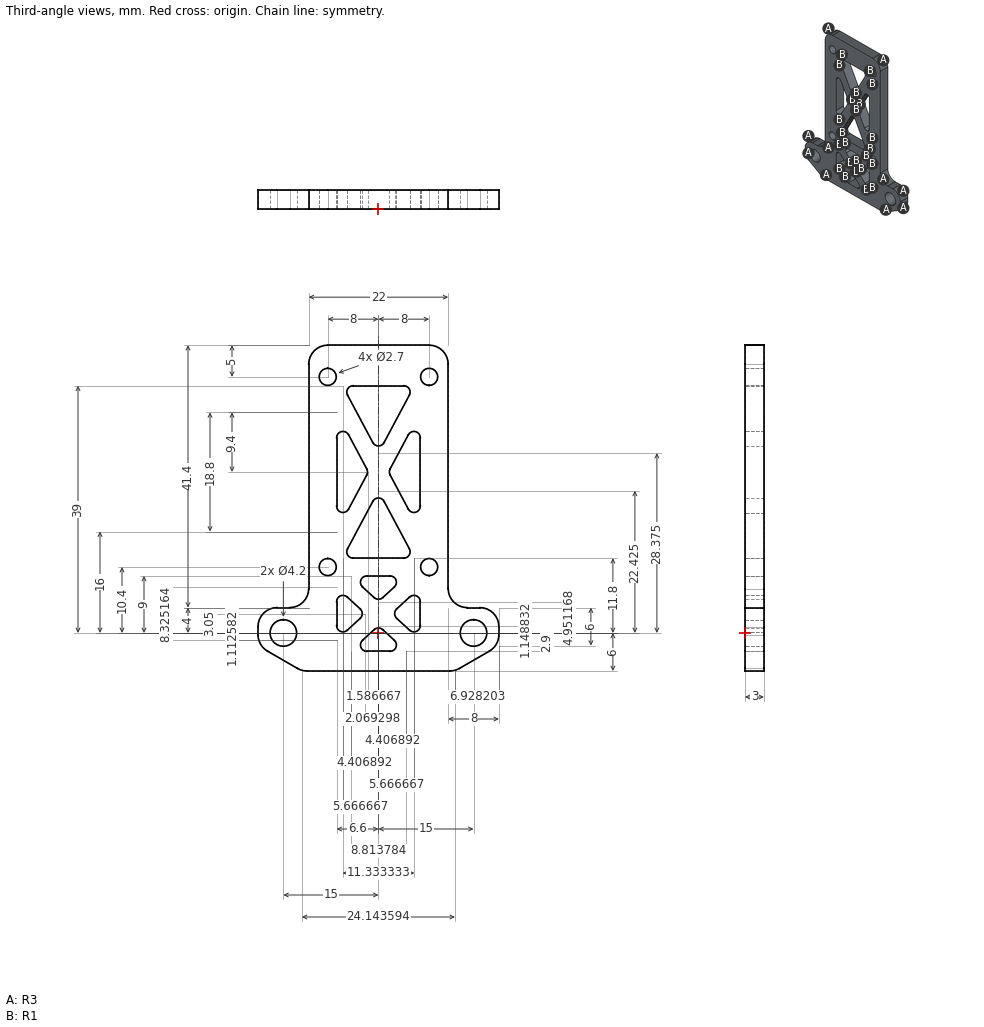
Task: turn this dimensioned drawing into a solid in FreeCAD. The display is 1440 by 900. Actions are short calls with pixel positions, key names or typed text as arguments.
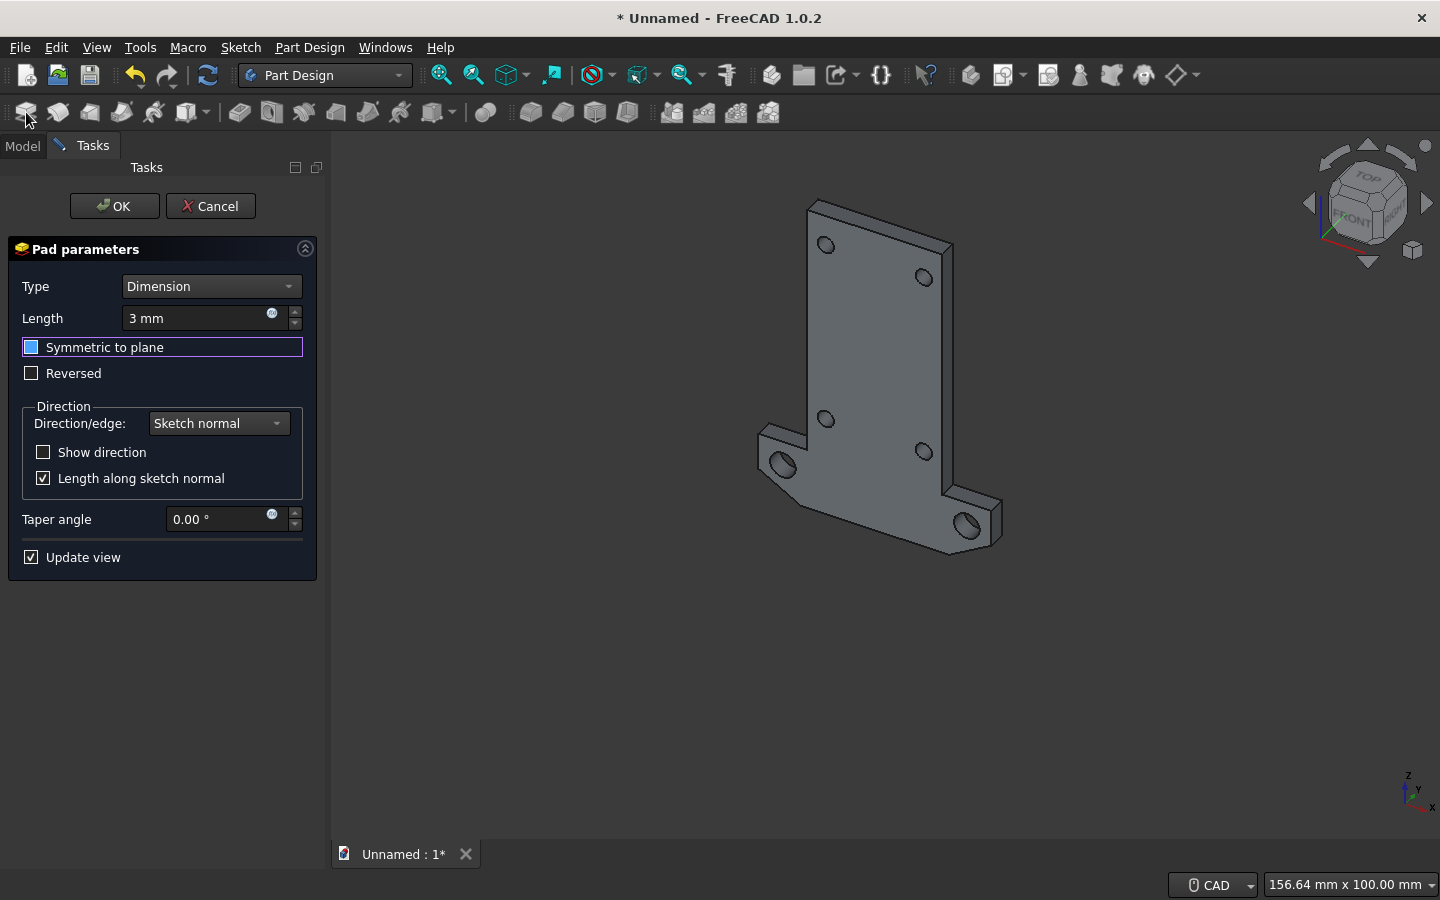
click(30, 373)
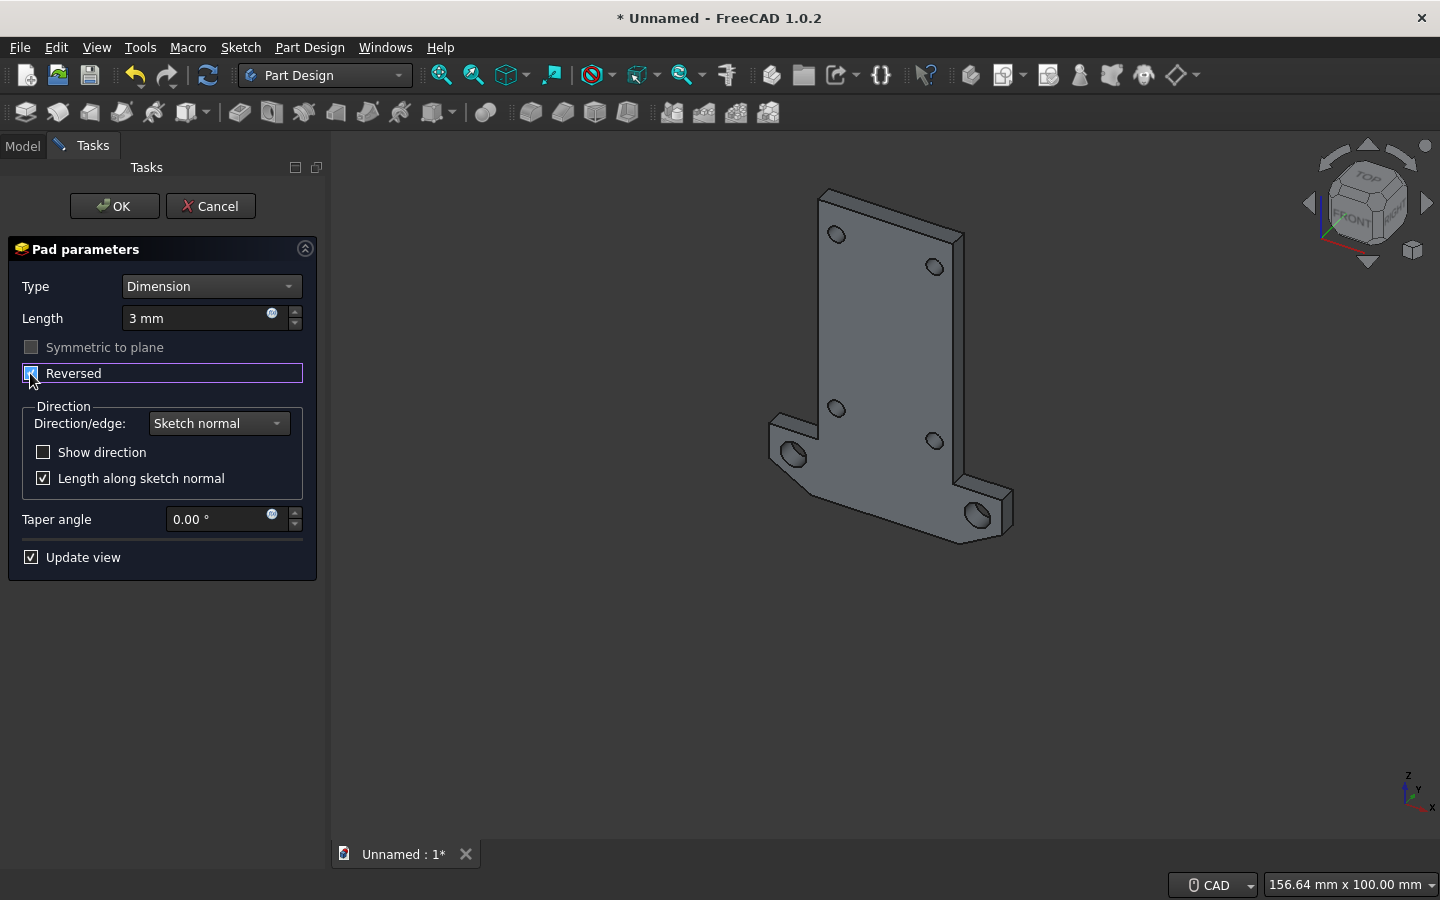
click(115, 206)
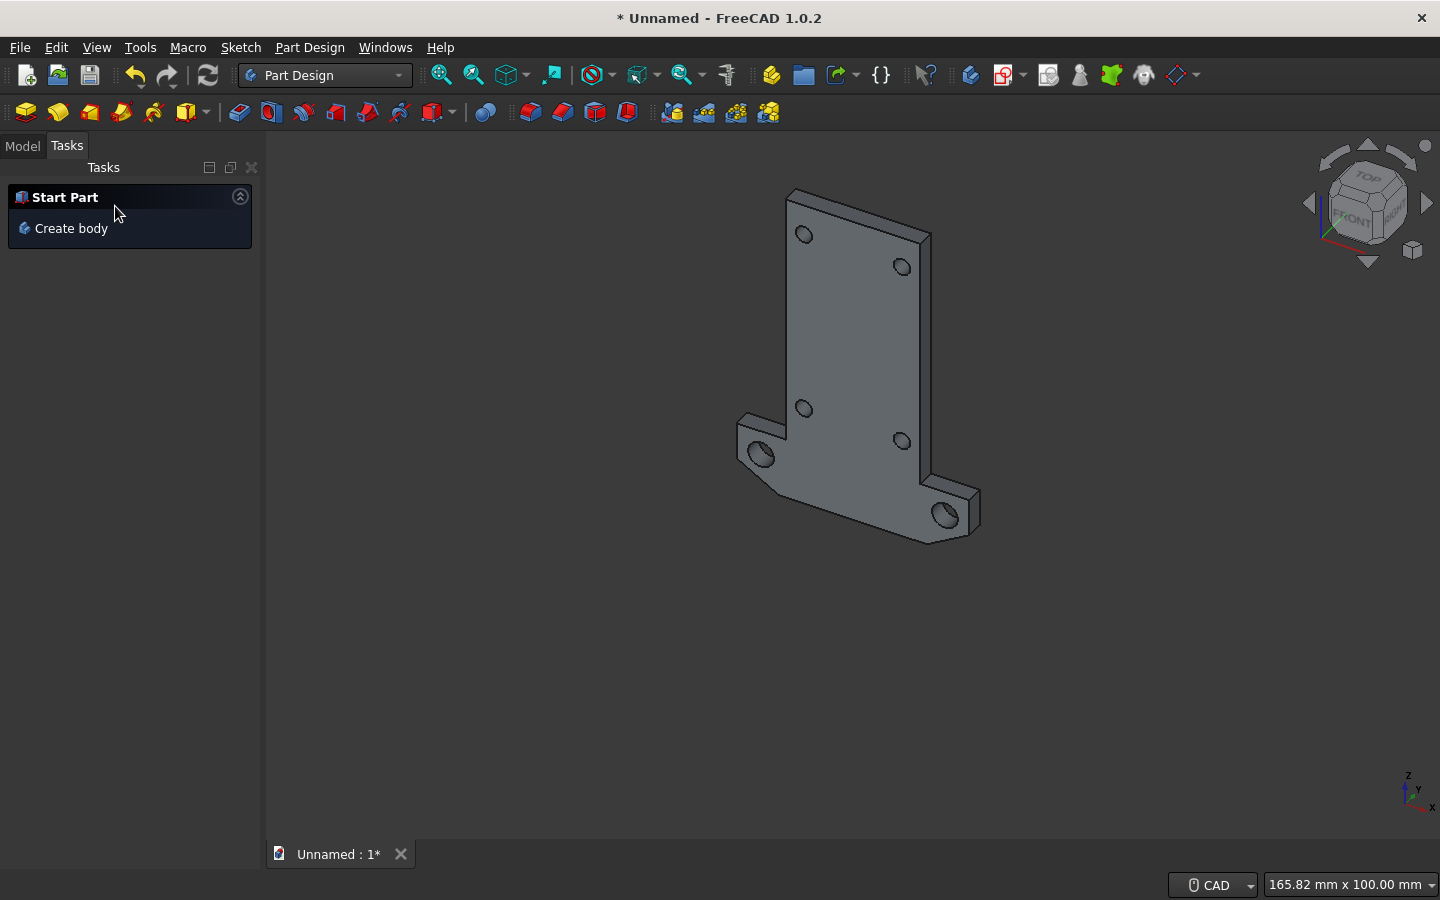
key(4)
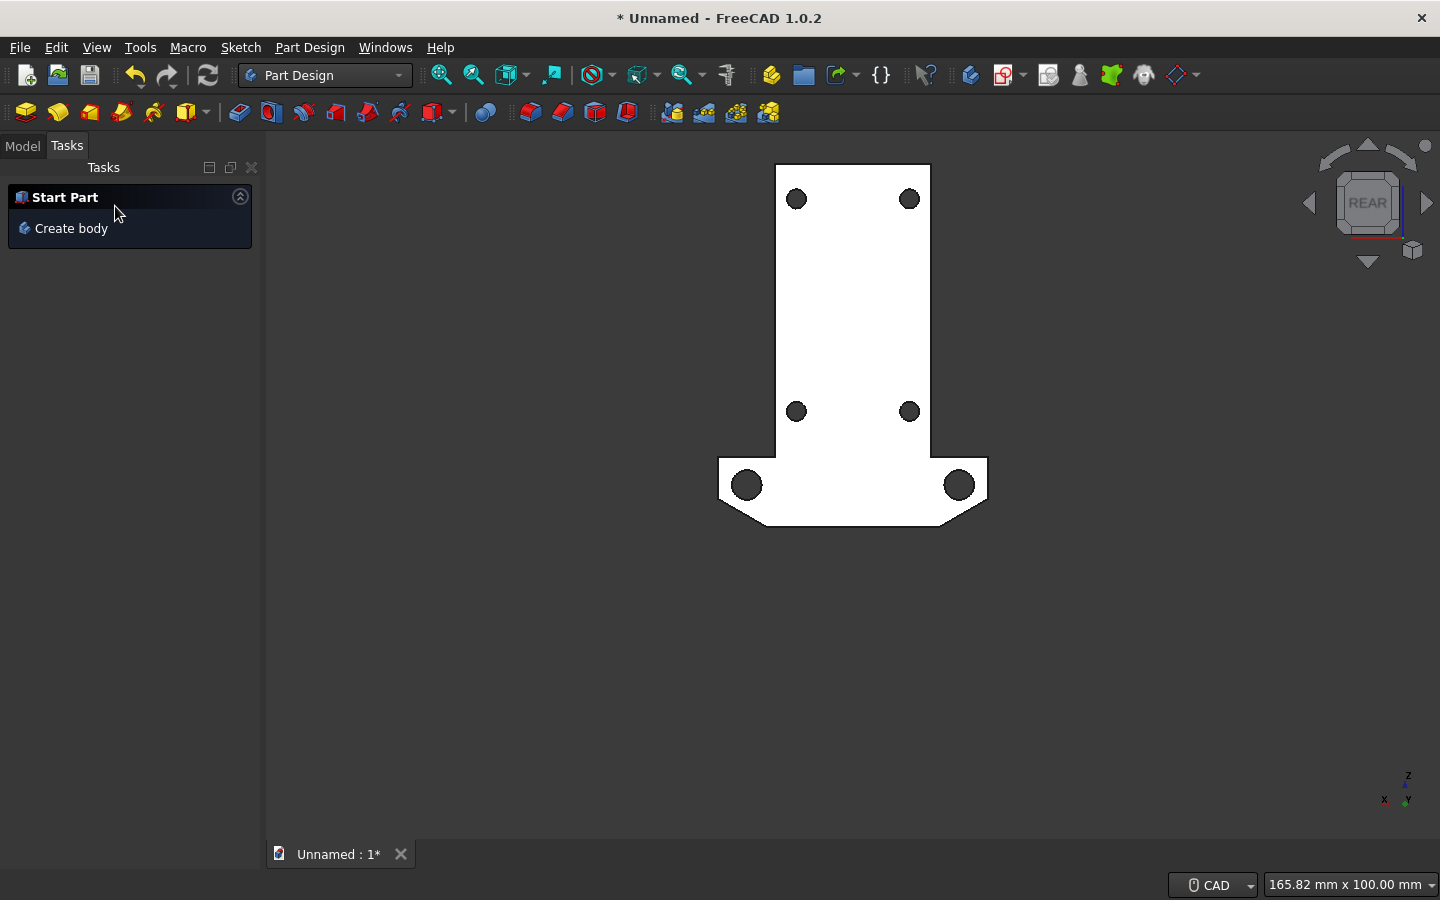
click(853, 293)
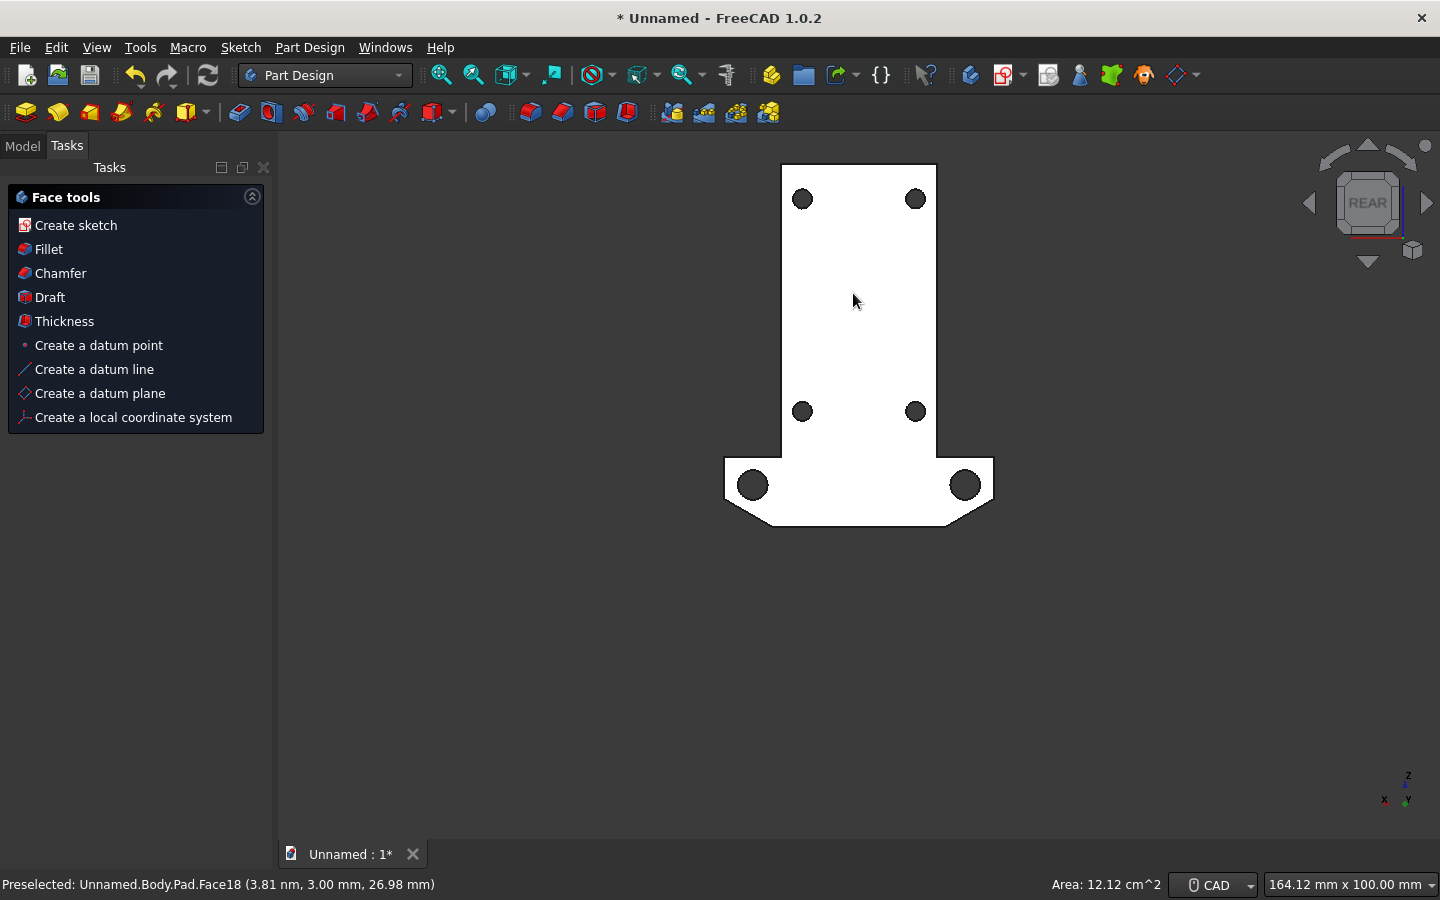
click(1004, 76)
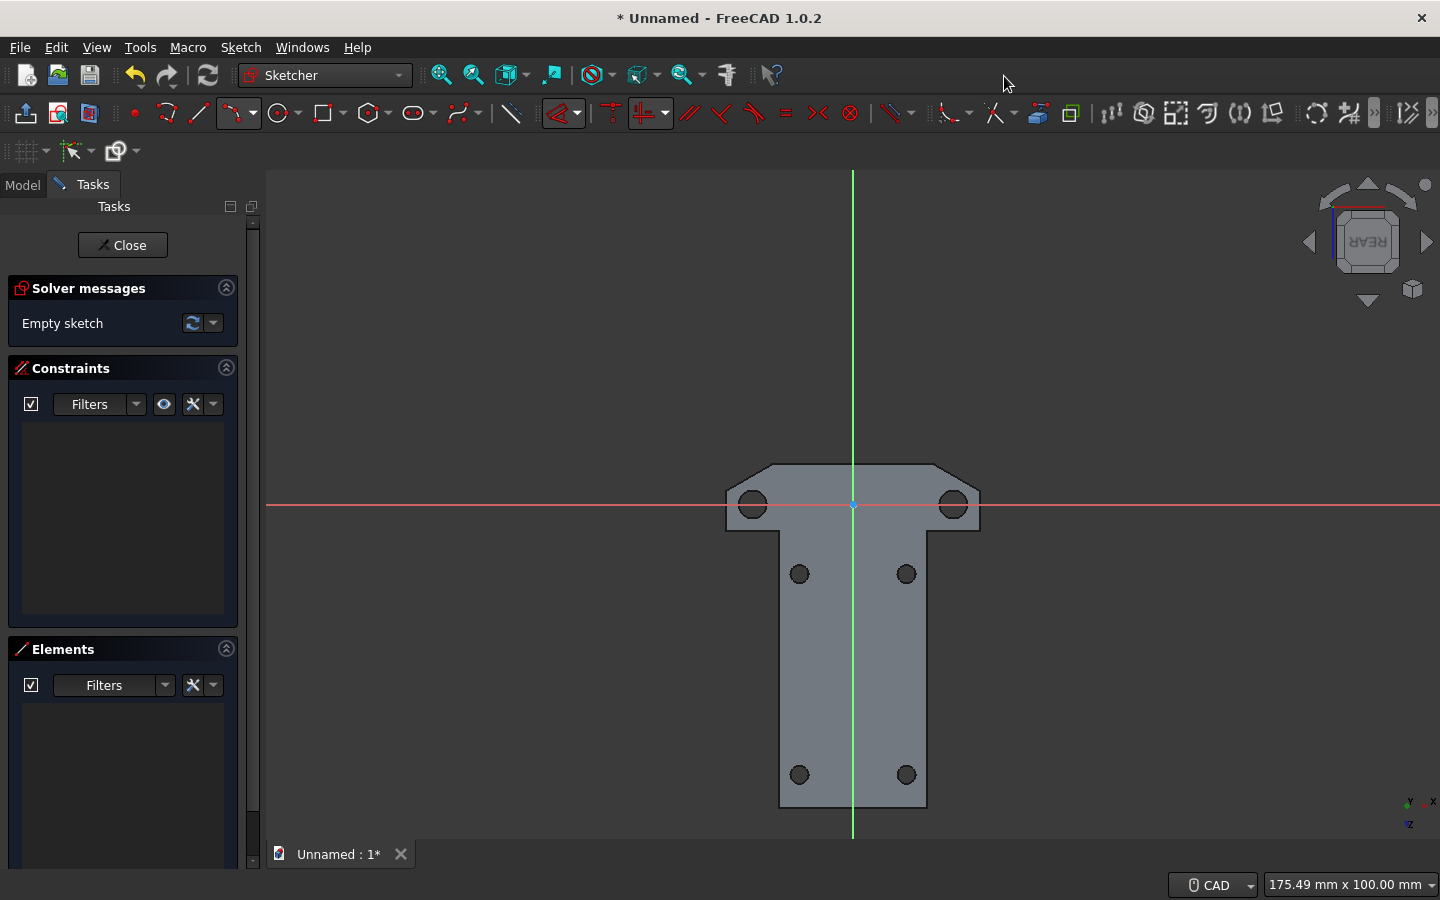
scroll(992, 811, up, 2)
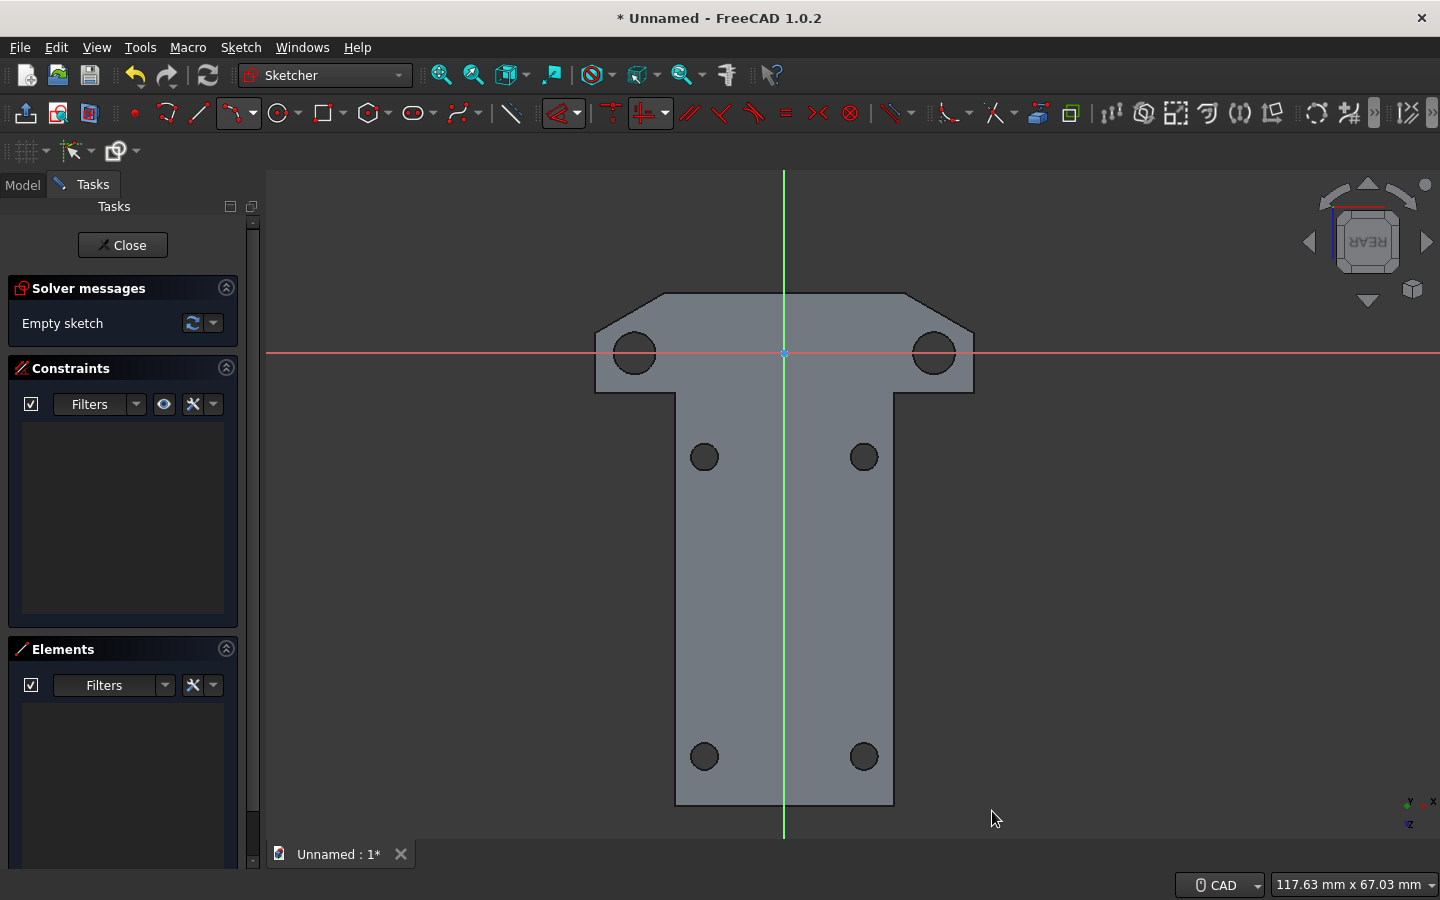
key(g)
key(m)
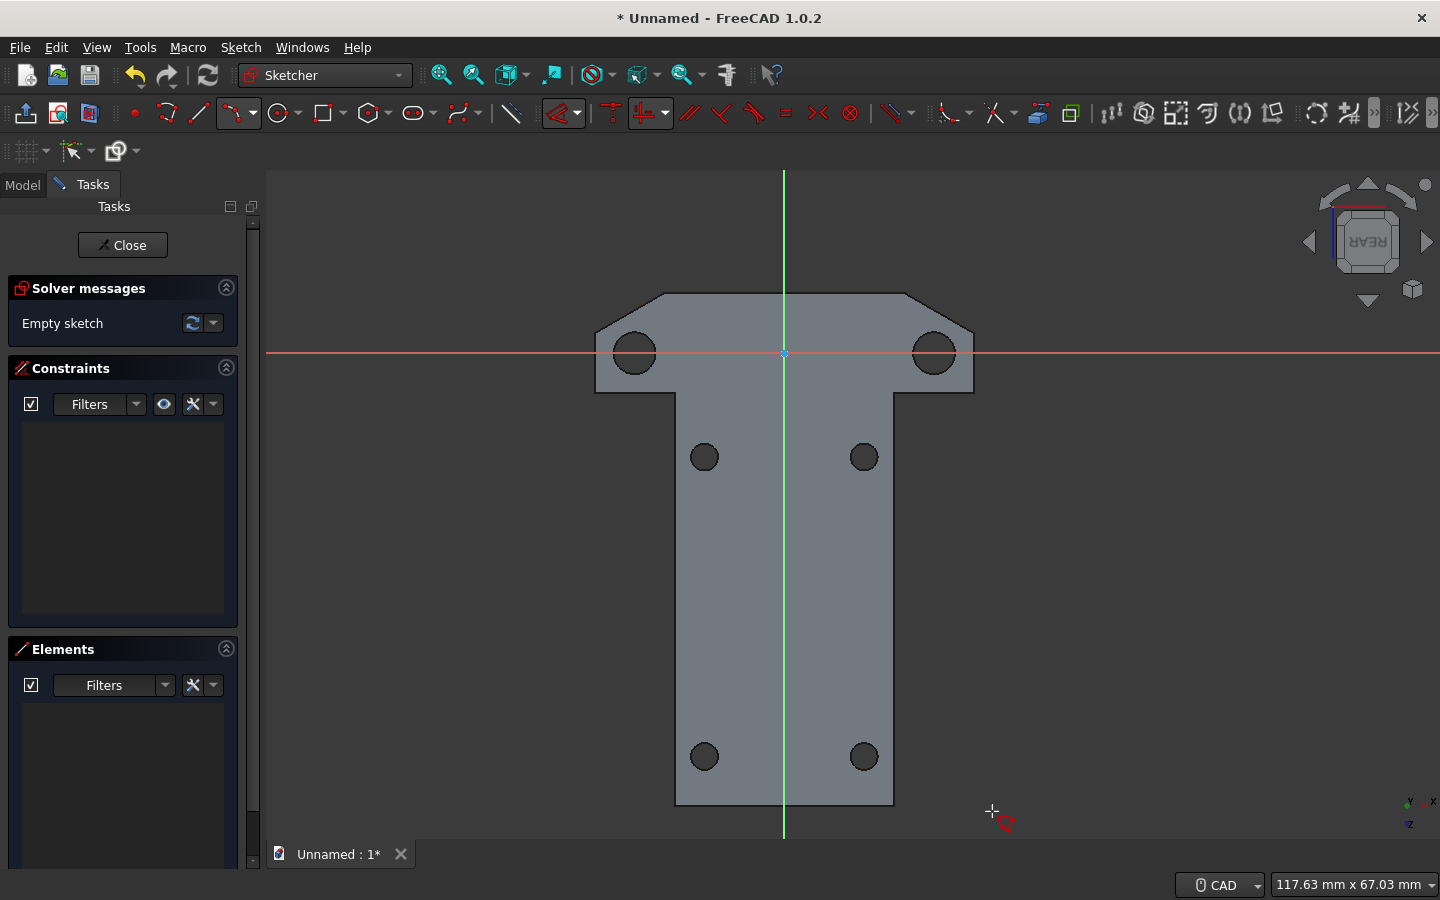
click(764, 384)